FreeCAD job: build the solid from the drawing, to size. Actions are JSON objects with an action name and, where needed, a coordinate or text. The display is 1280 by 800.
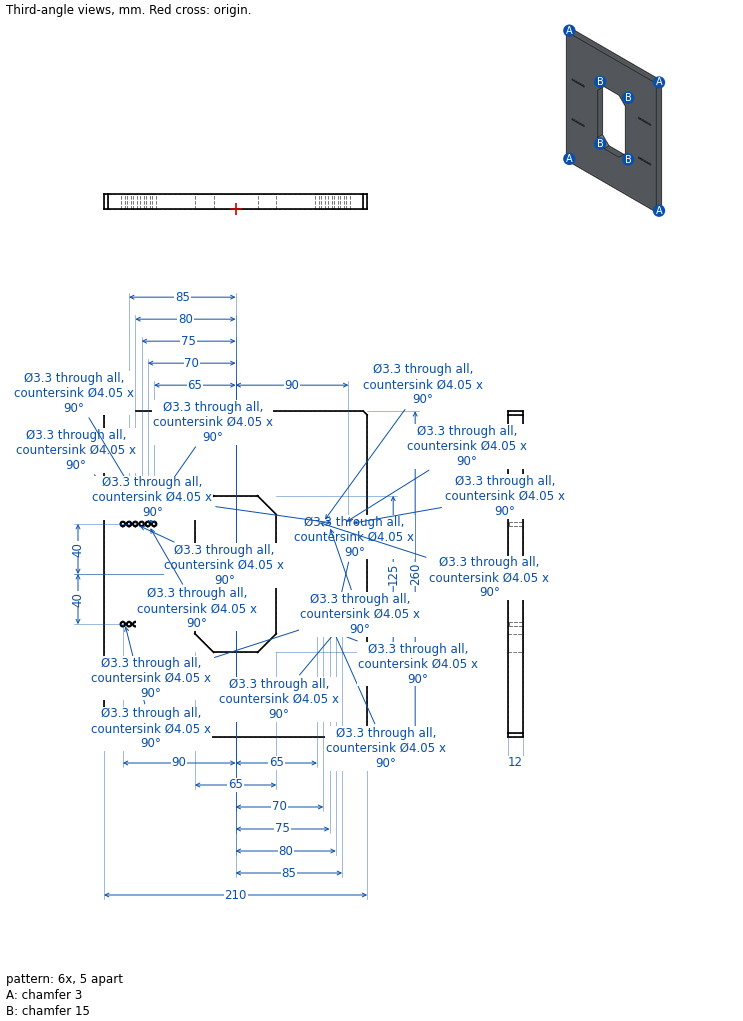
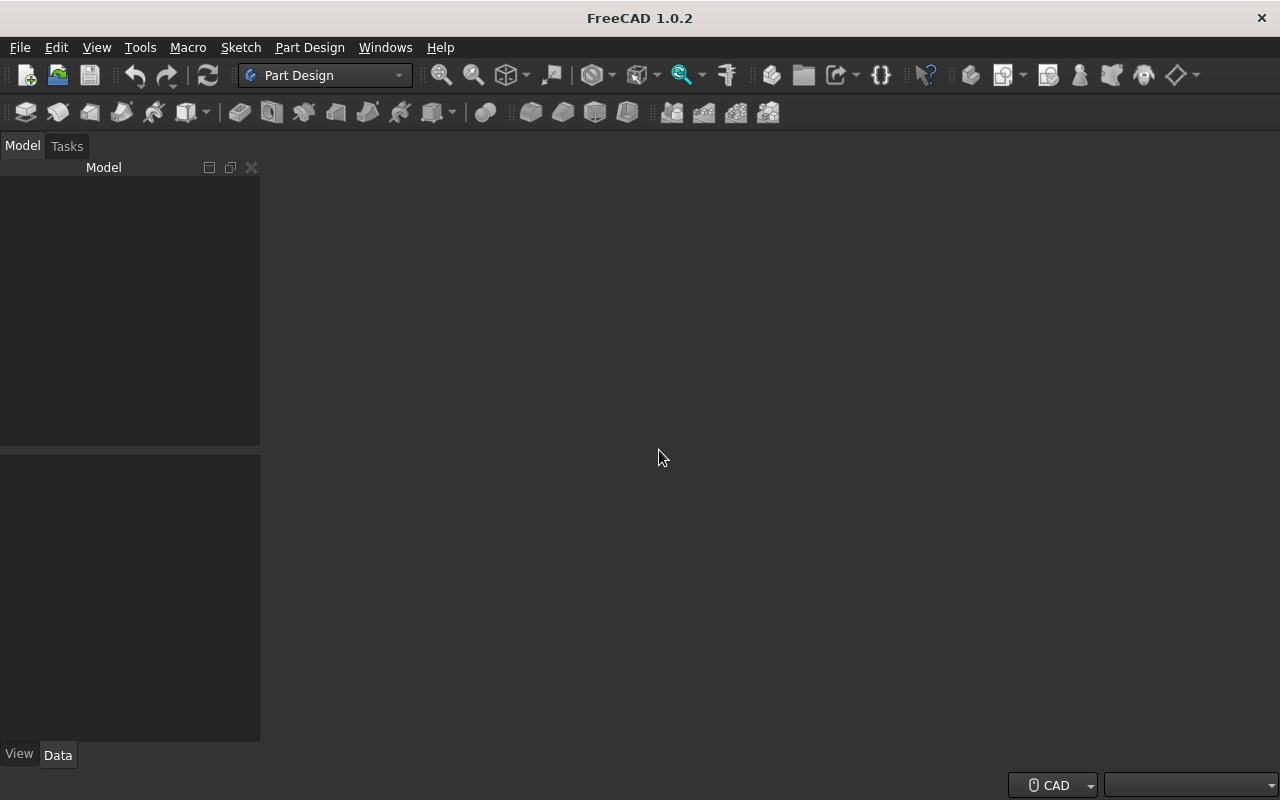
{"action": "left_click", "coordinate": [26, 76]}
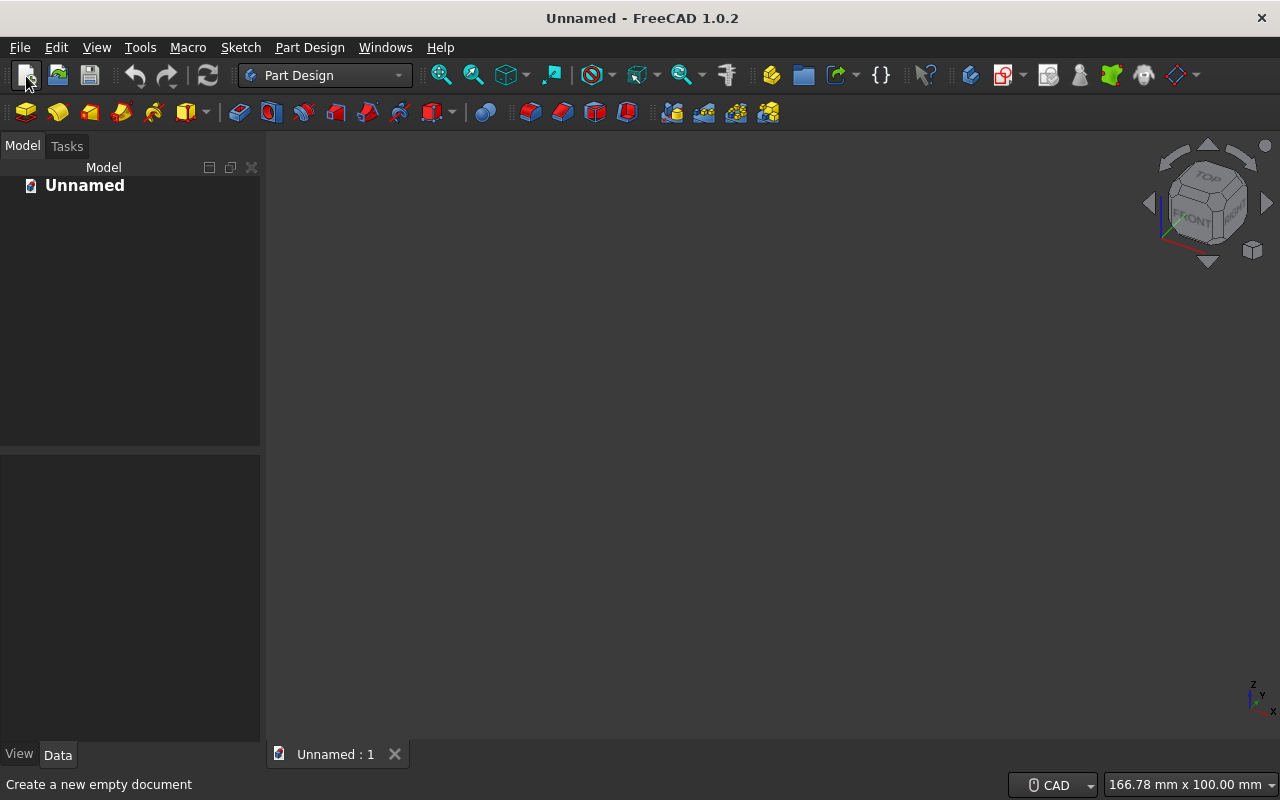
{"action": "left_click", "coordinate": [1004, 76]}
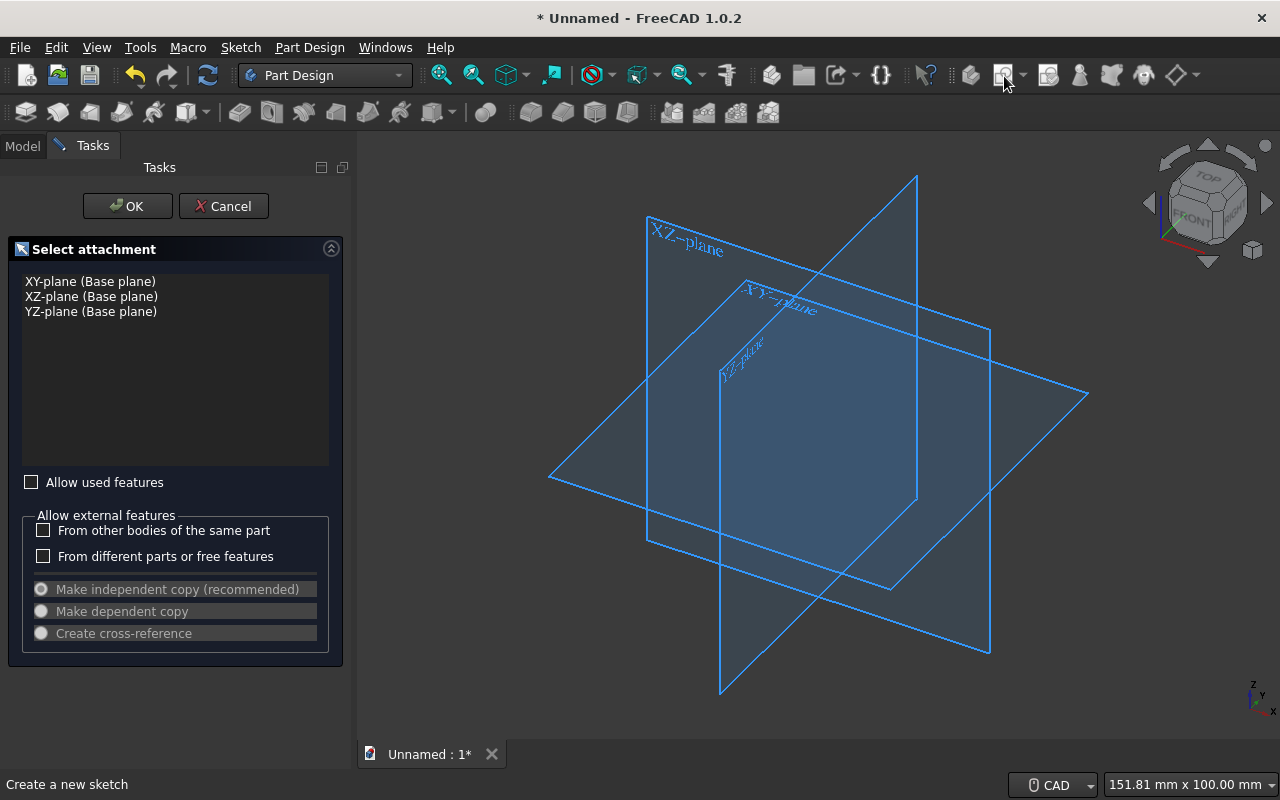
{"action": "left_click", "coordinate": [82, 296]}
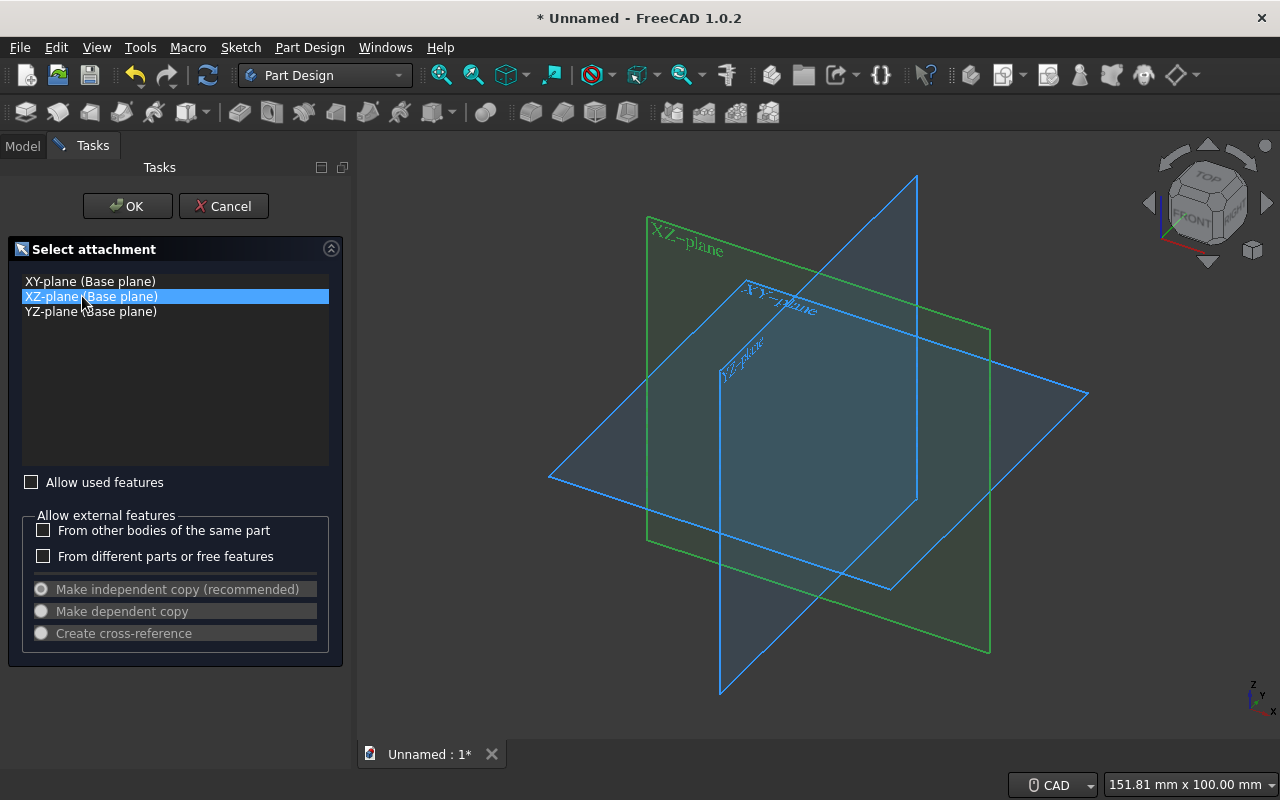
{"action": "left_click", "coordinate": [128, 206]}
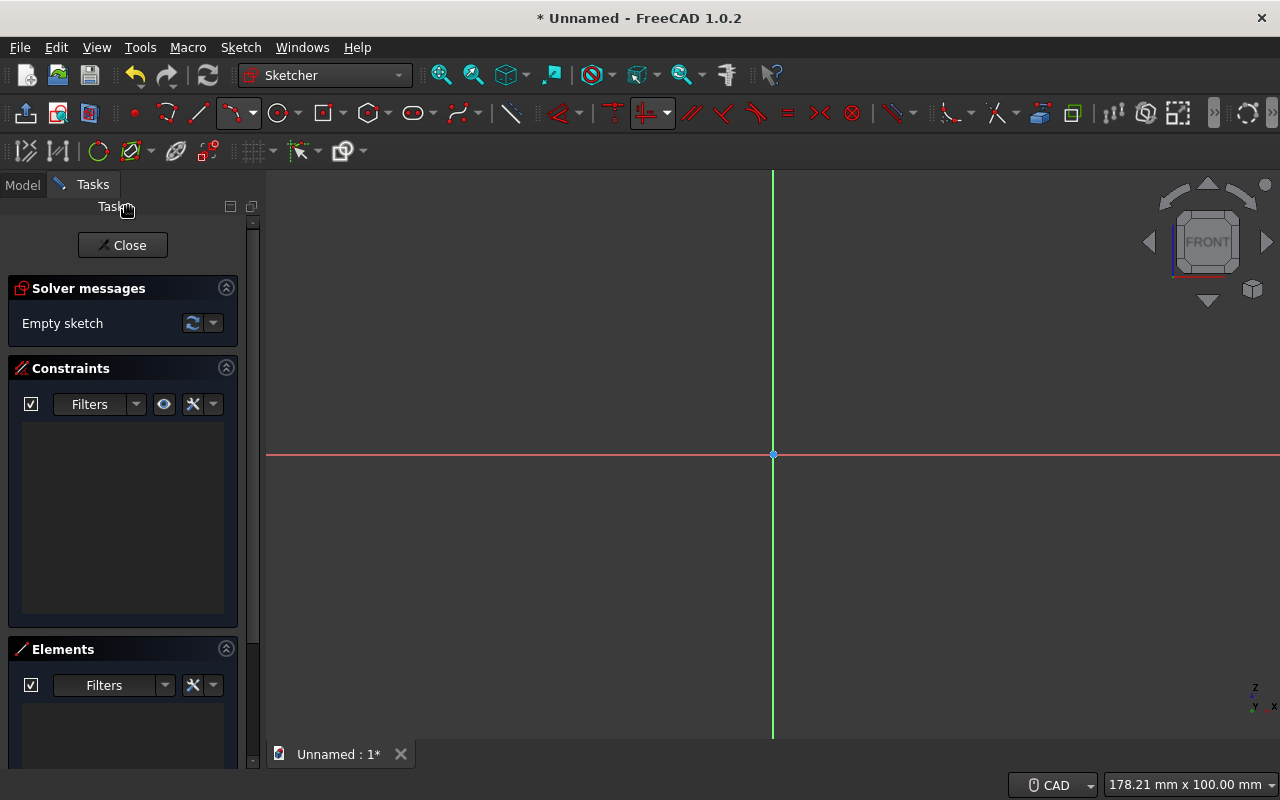
{"action": "scroll", "coordinate": [682, 454], "scroll_direction": "down", "scroll_amount": 7}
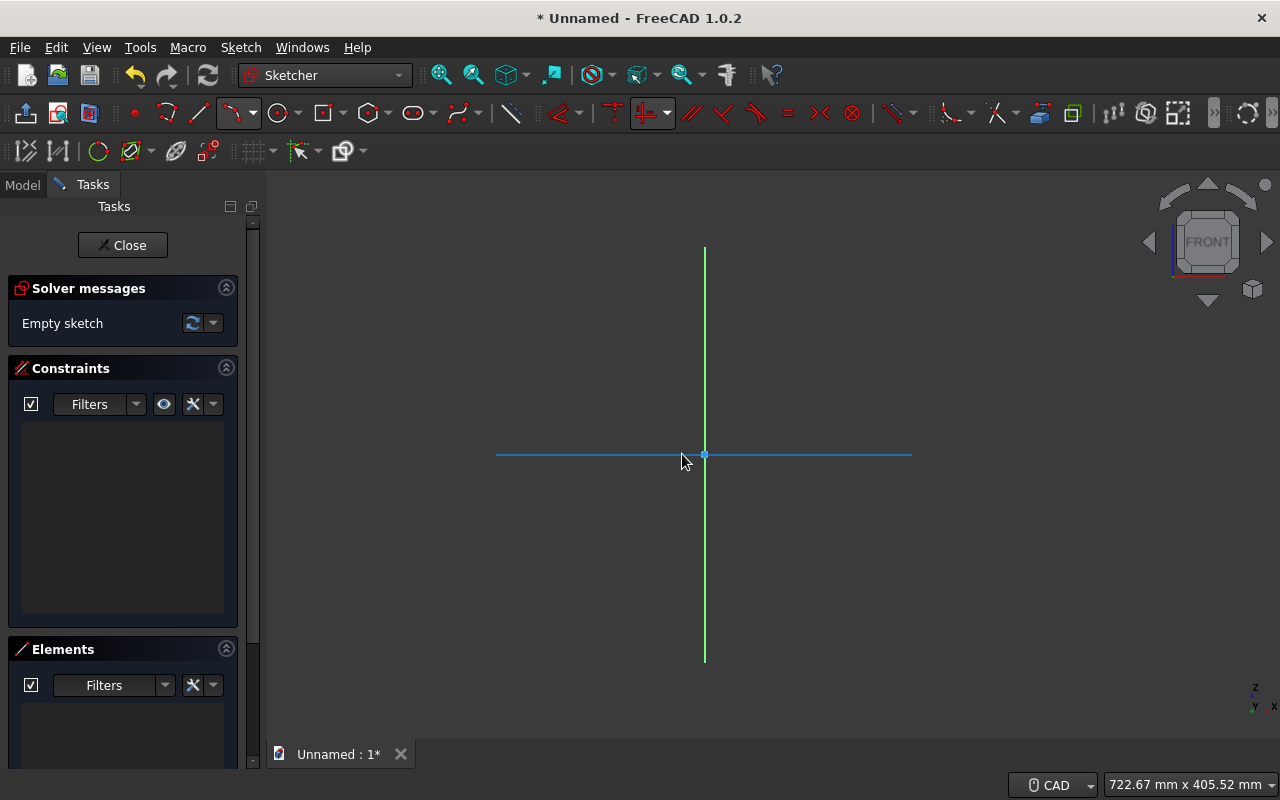
{"action": "left_click", "coordinate": [324, 114]}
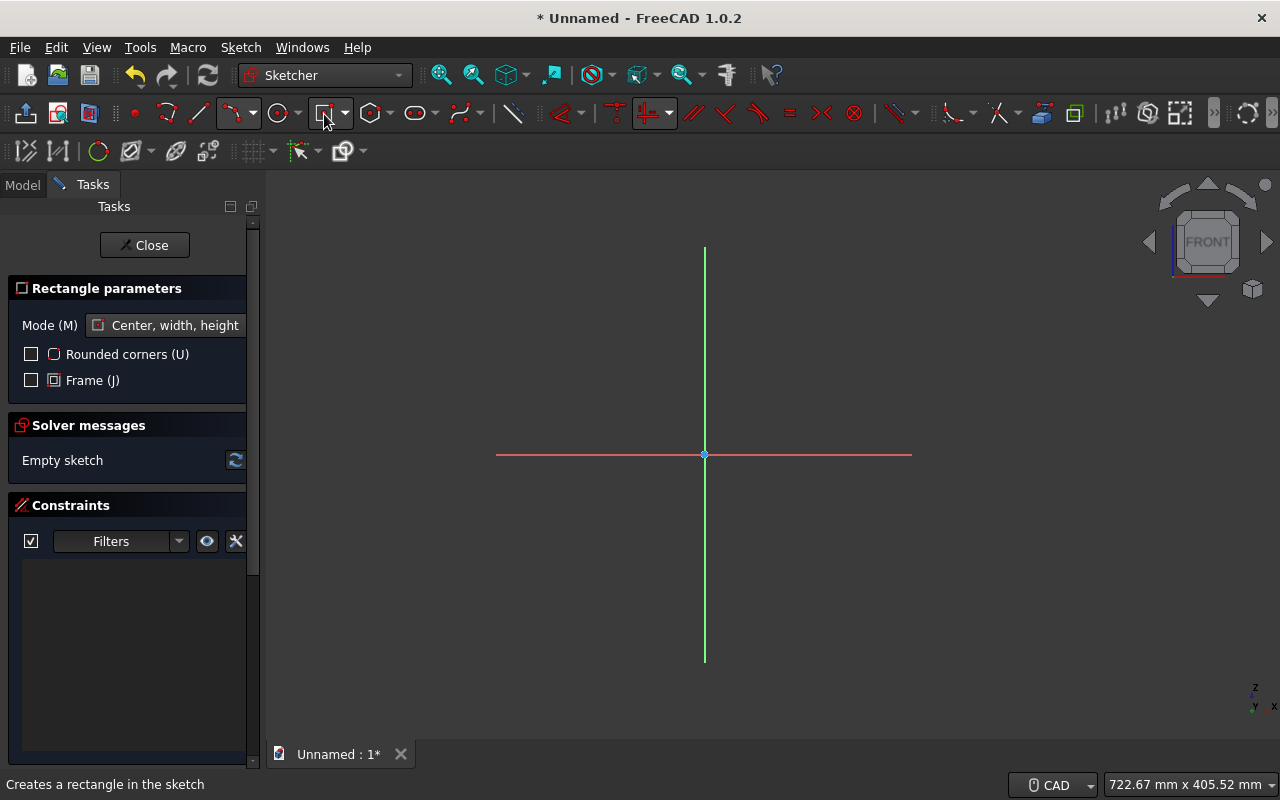
{"action": "left_click", "coordinate": [705, 454]}
{"action": "mouse_move", "coordinate": [852, 272]}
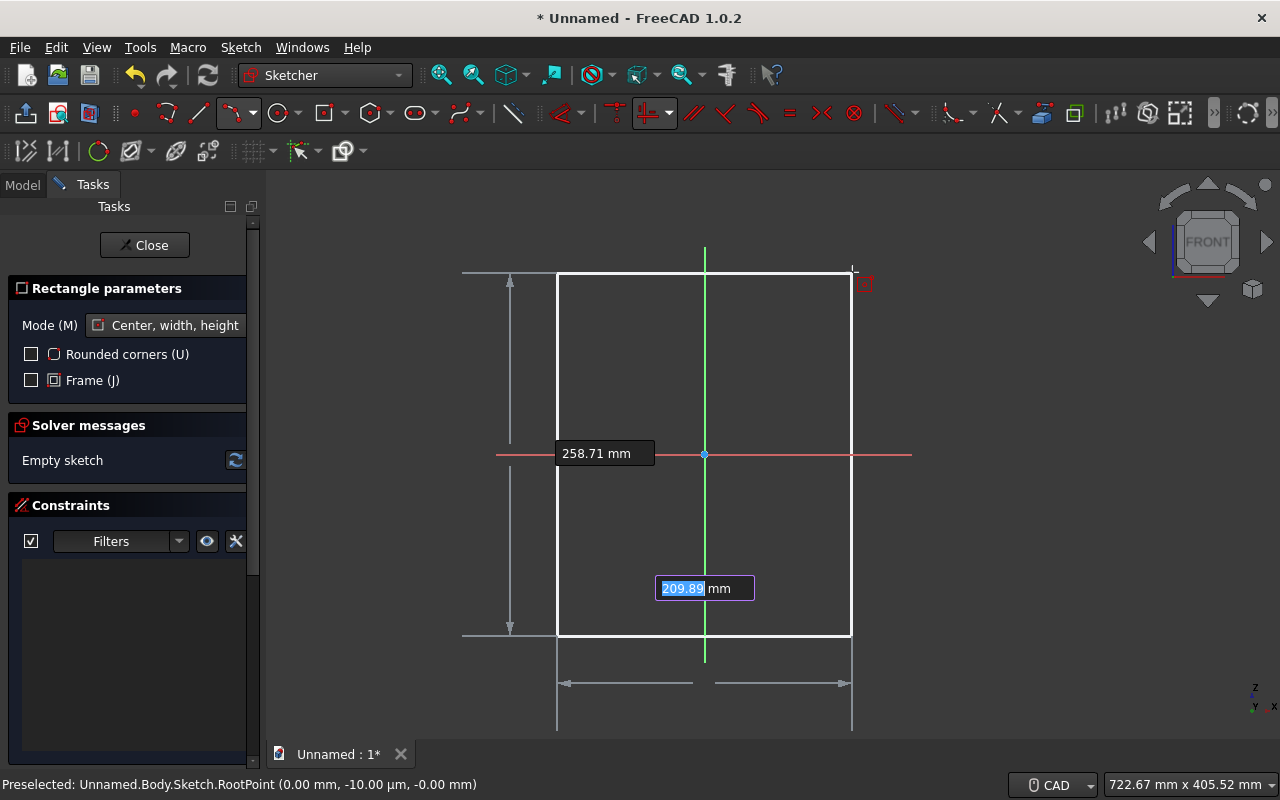
{"action": "type", "text": "210"}
{"action": "key", "text": "Tab"}
{"action": "type", "text": "260"}
{"action": "key", "text": "Return"}
{"action": "key", "text": "Escape"}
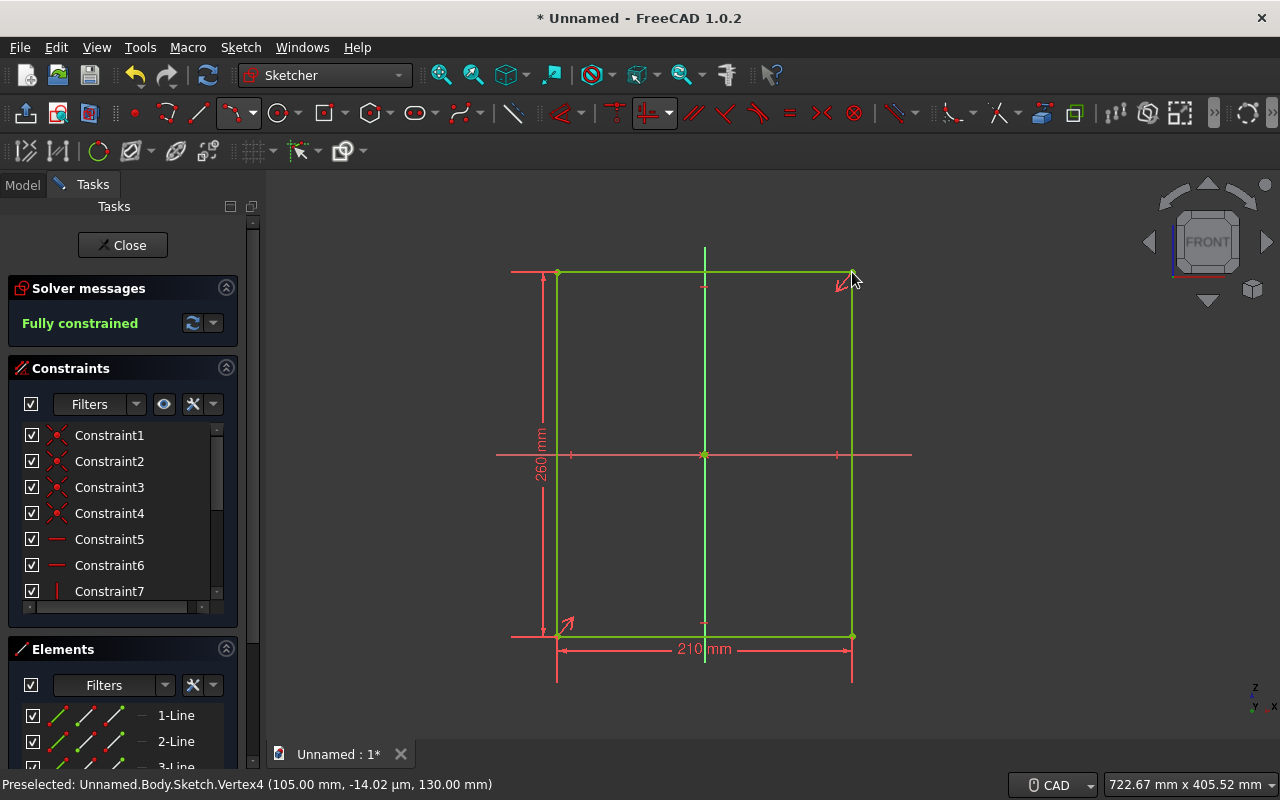
{"action": "left_click", "coordinate": [123, 245]}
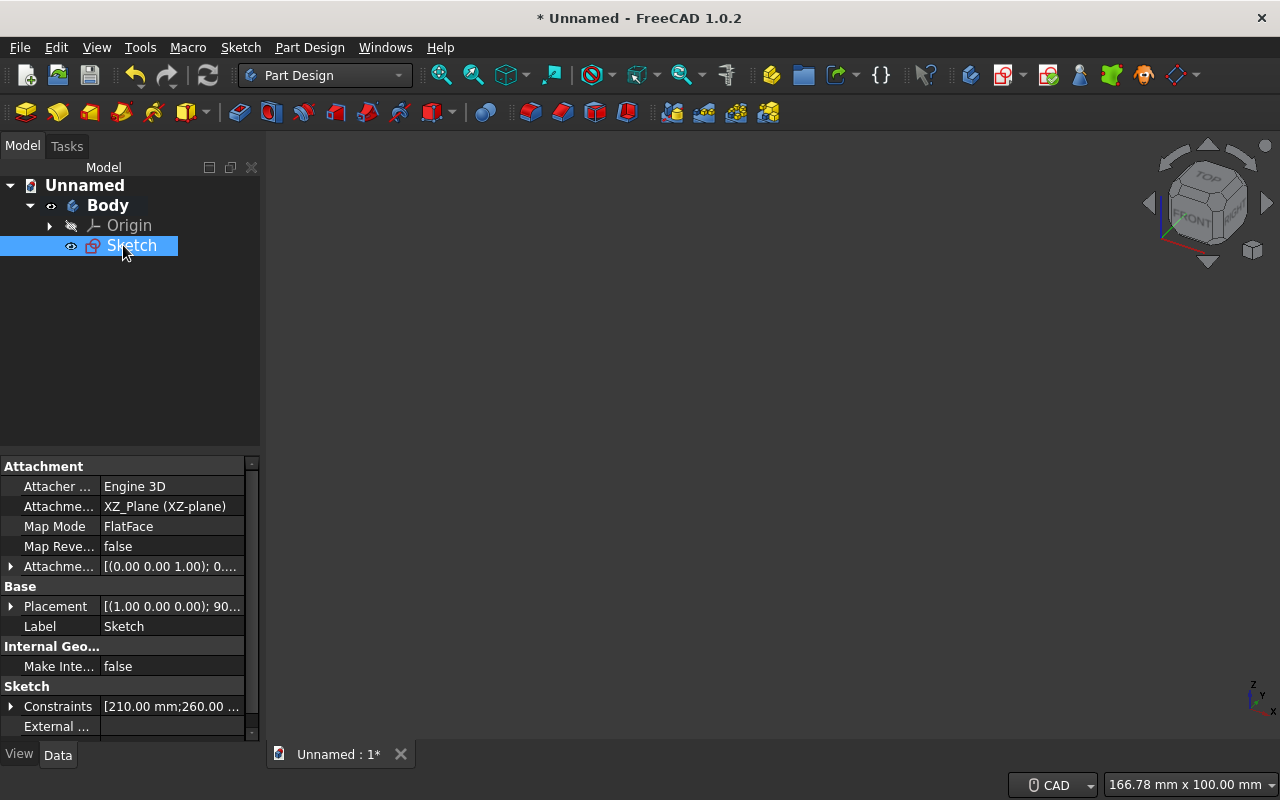
{"action": "left_click", "coordinate": [26, 112]}